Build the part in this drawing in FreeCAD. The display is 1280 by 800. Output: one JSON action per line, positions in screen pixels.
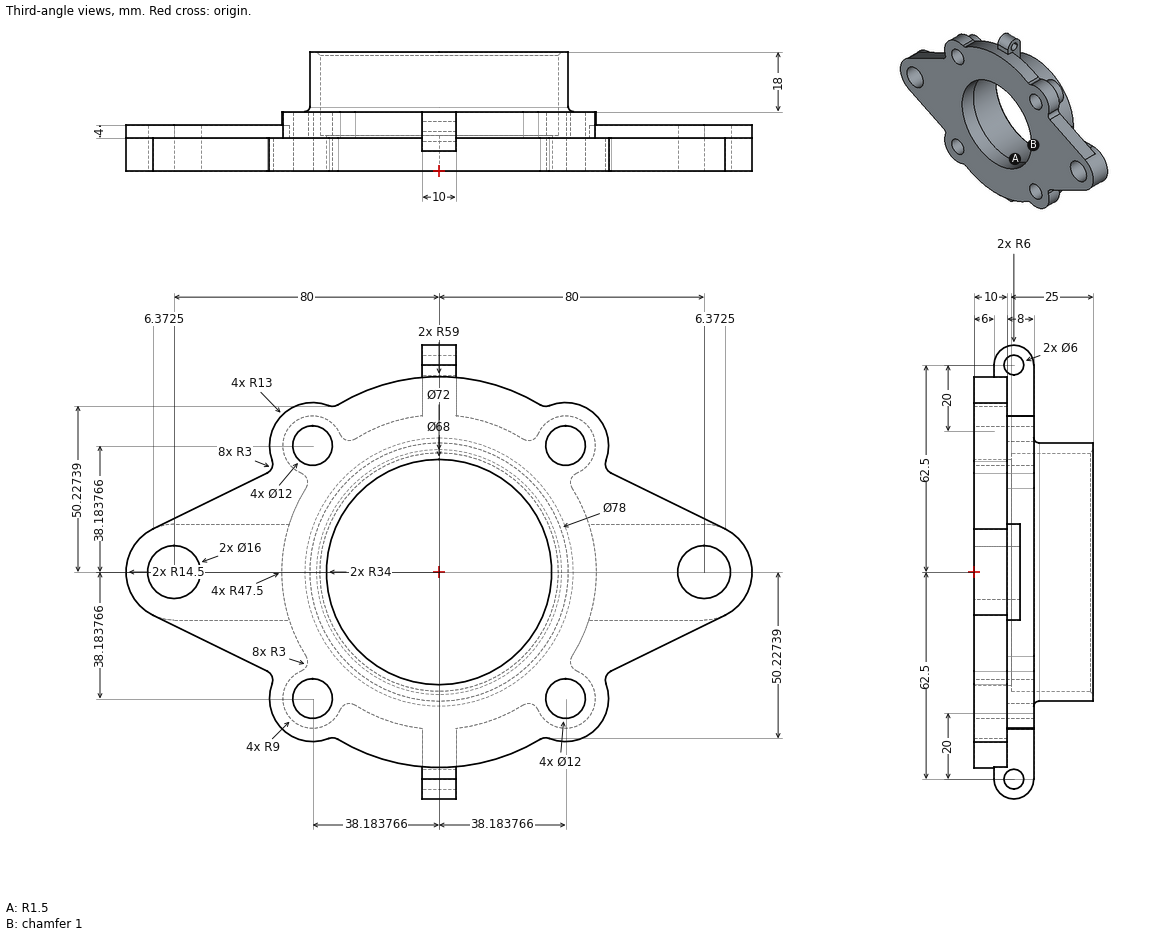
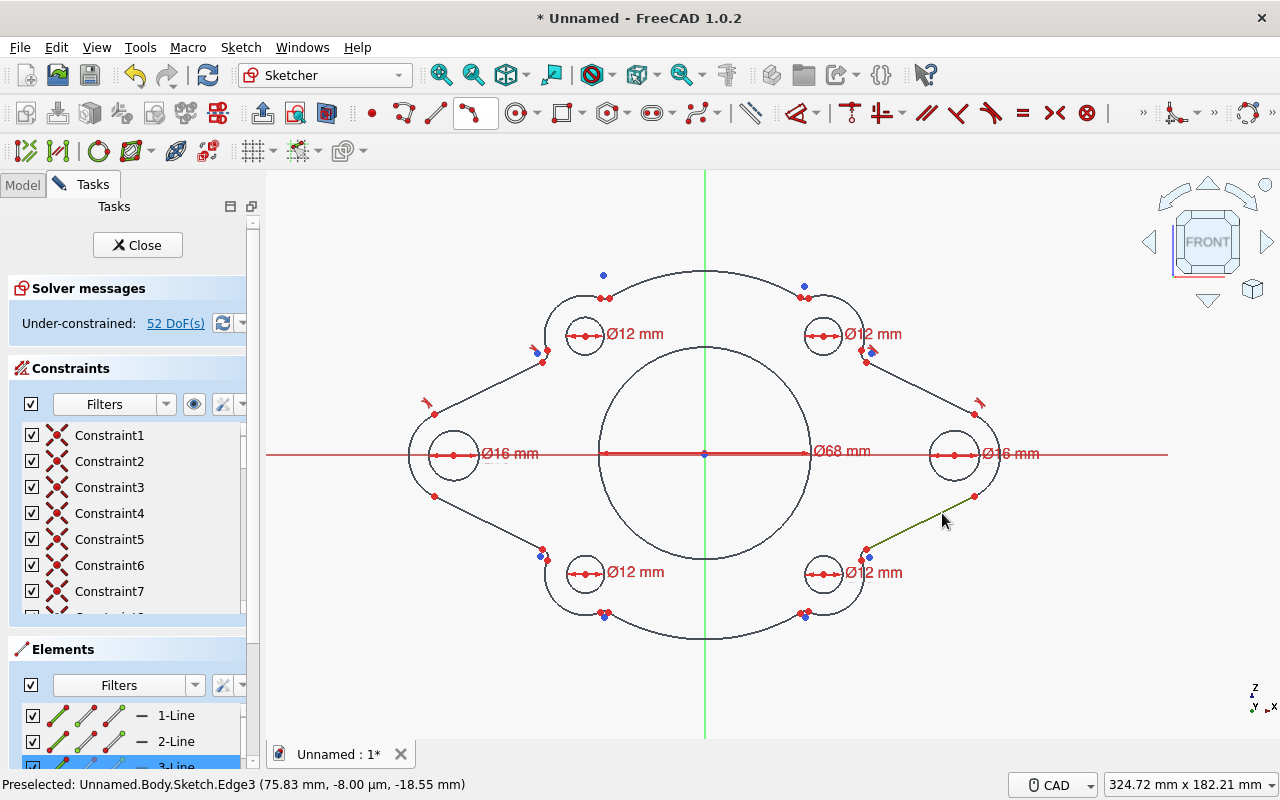
{"action": "left_click", "coordinate": [995, 476]}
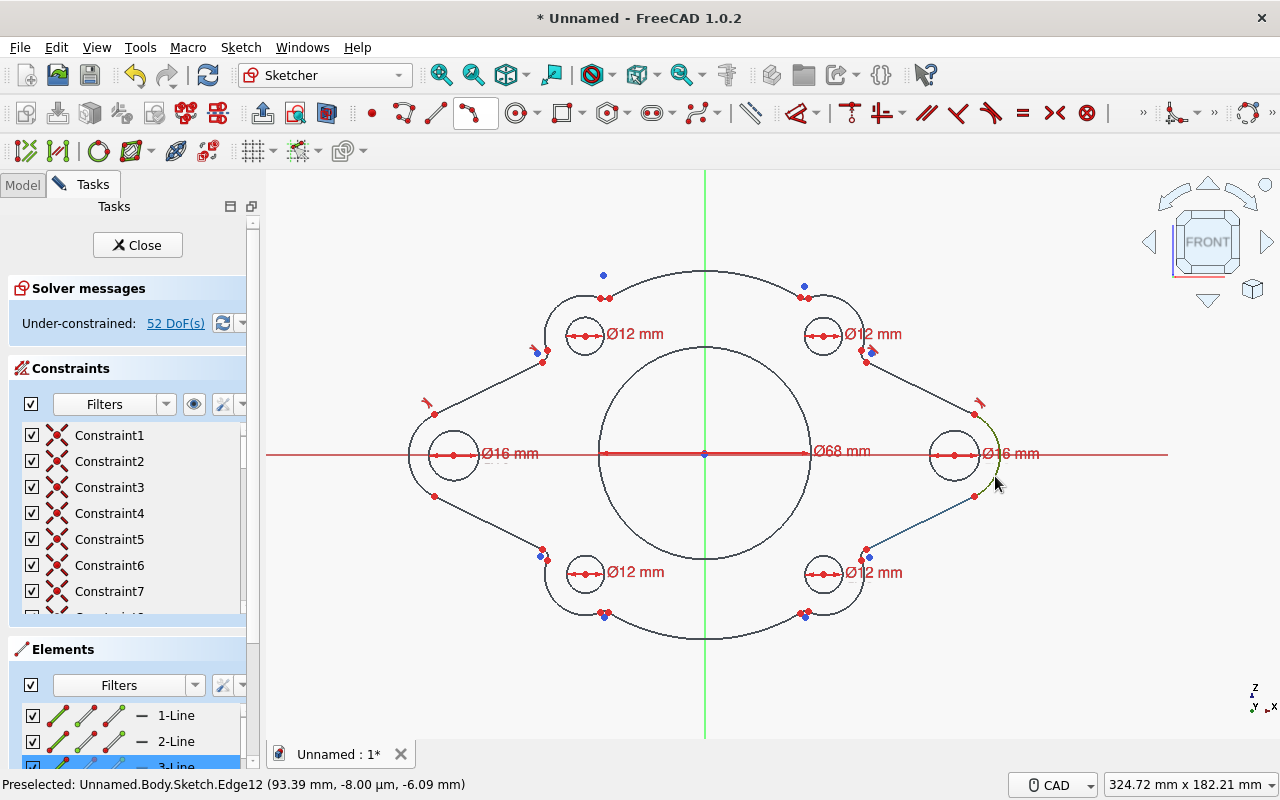
{"action": "left_click", "coordinate": [992, 114]}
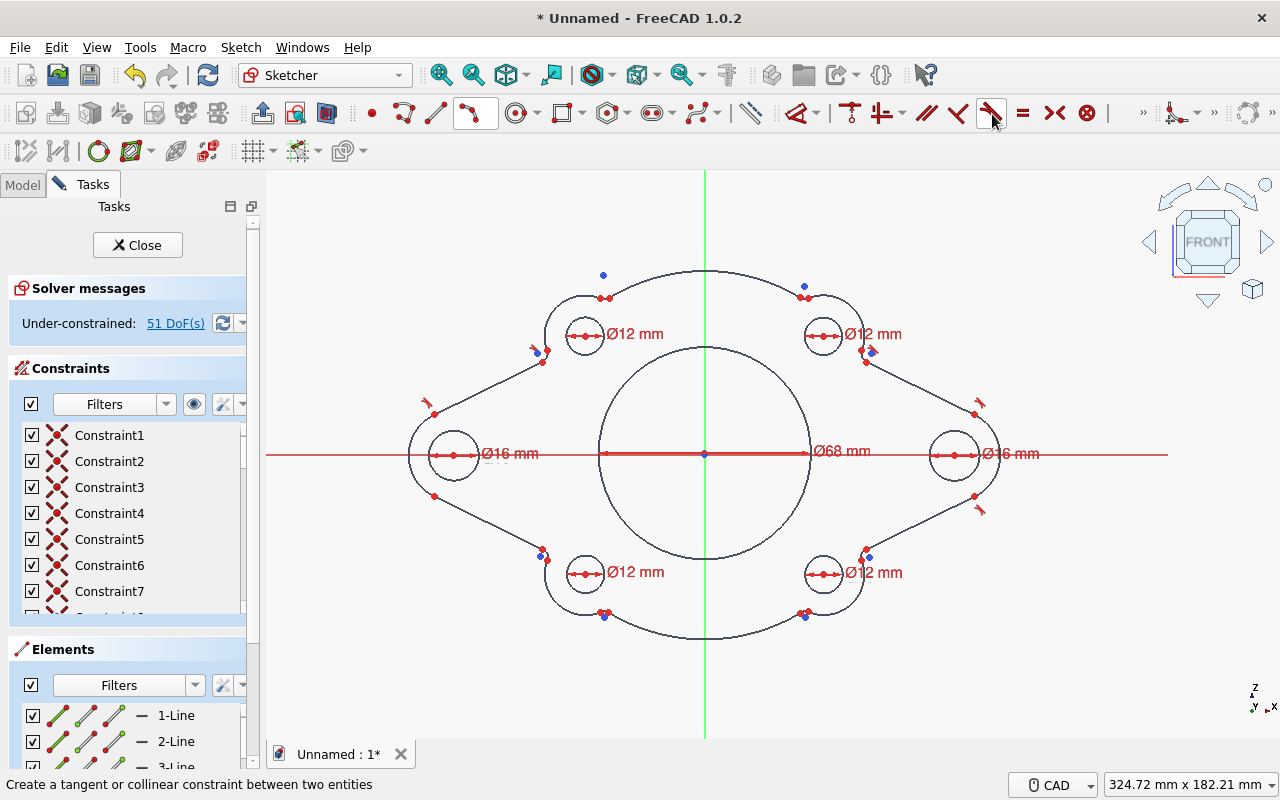
{"action": "left_click", "coordinate": [942, 513]}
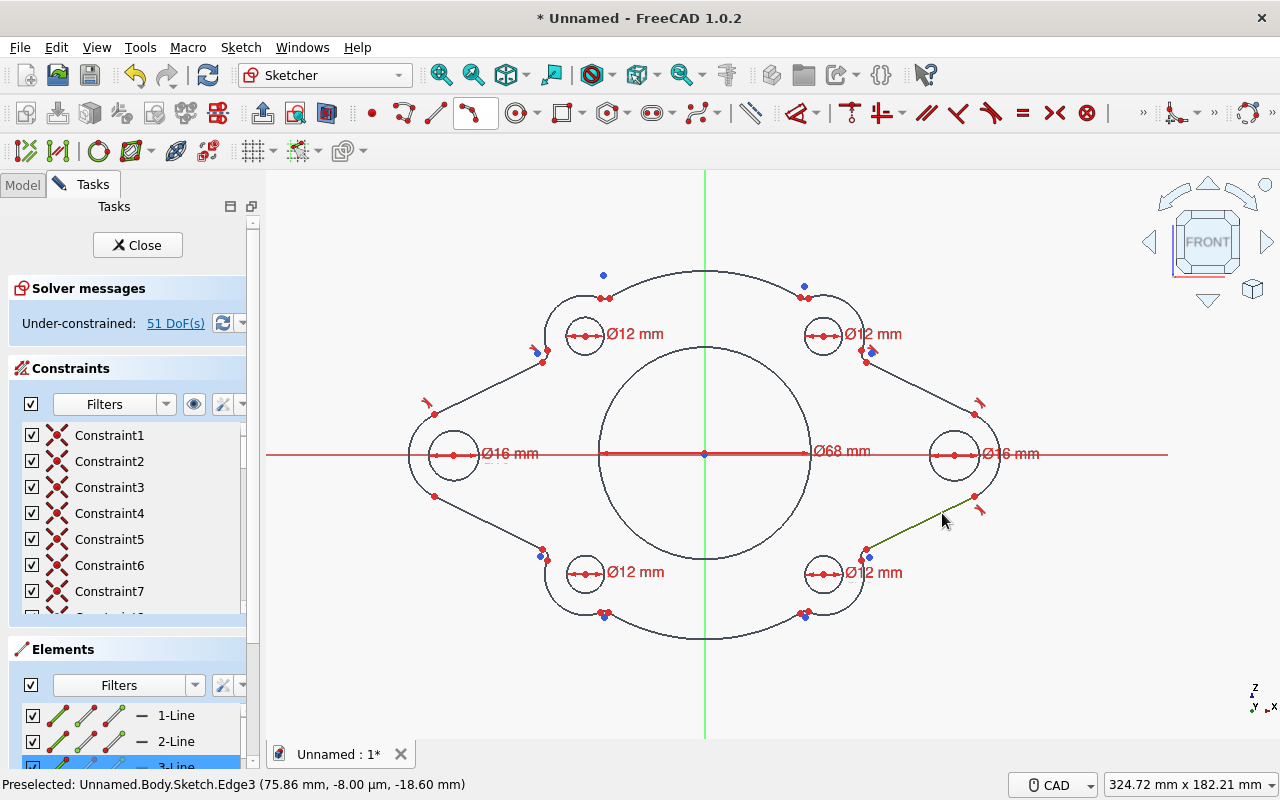
{"action": "scroll", "coordinate": [862, 554], "scroll_direction": "up", "scroll_amount": 4}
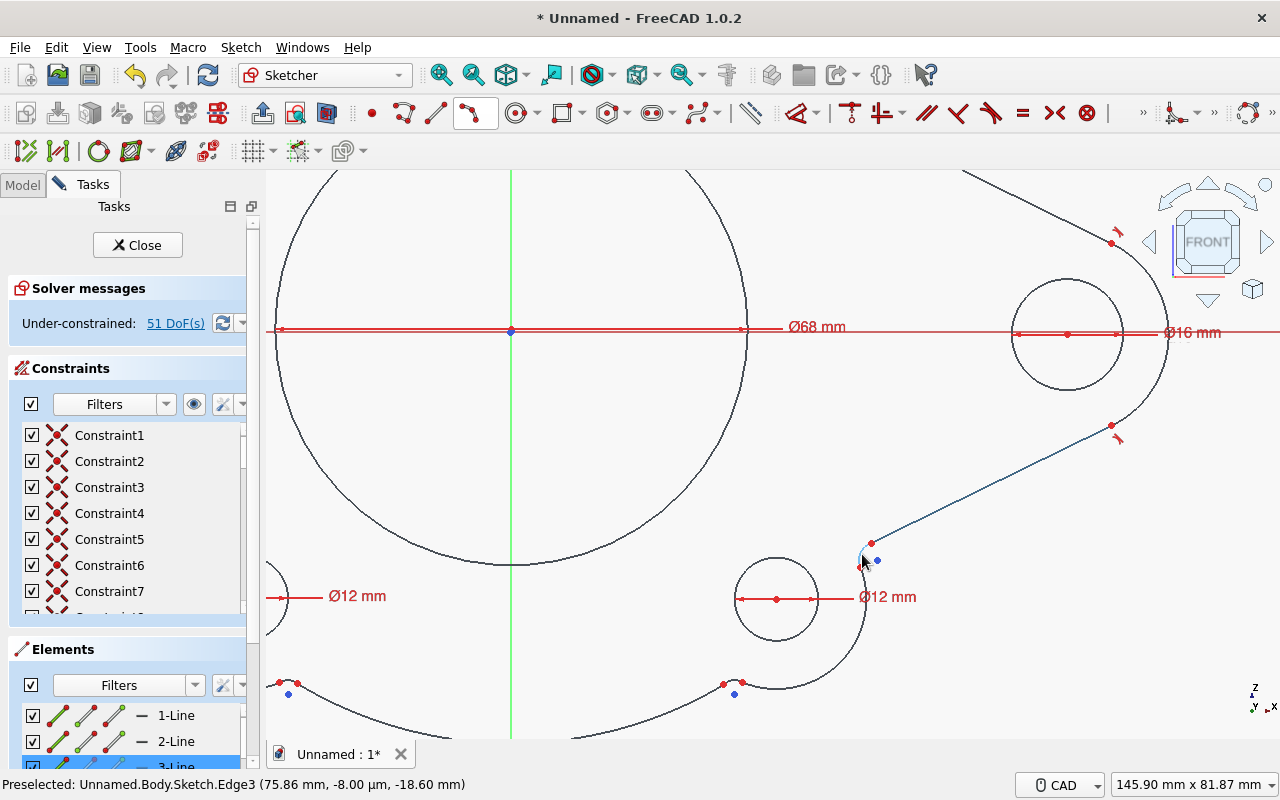
{"action": "left_click", "coordinate": [861, 553]}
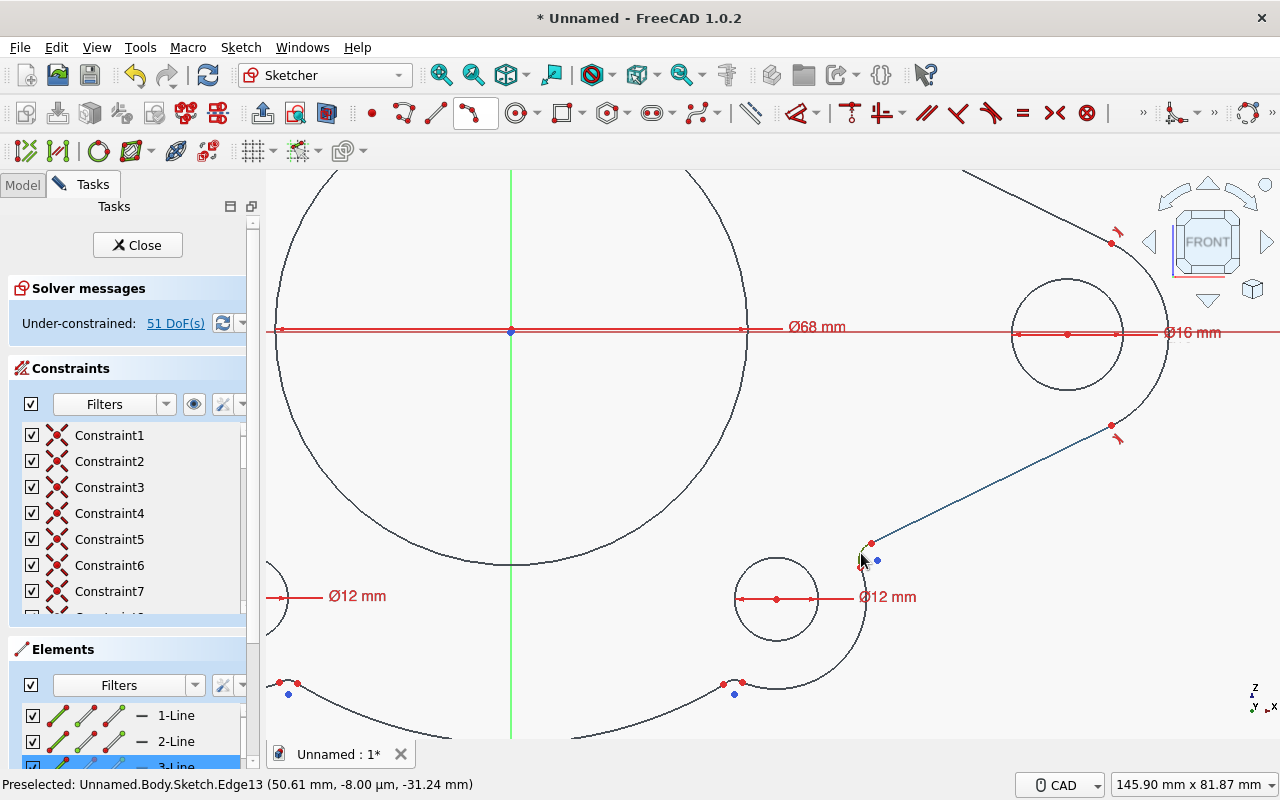
{"action": "left_click", "coordinate": [992, 114]}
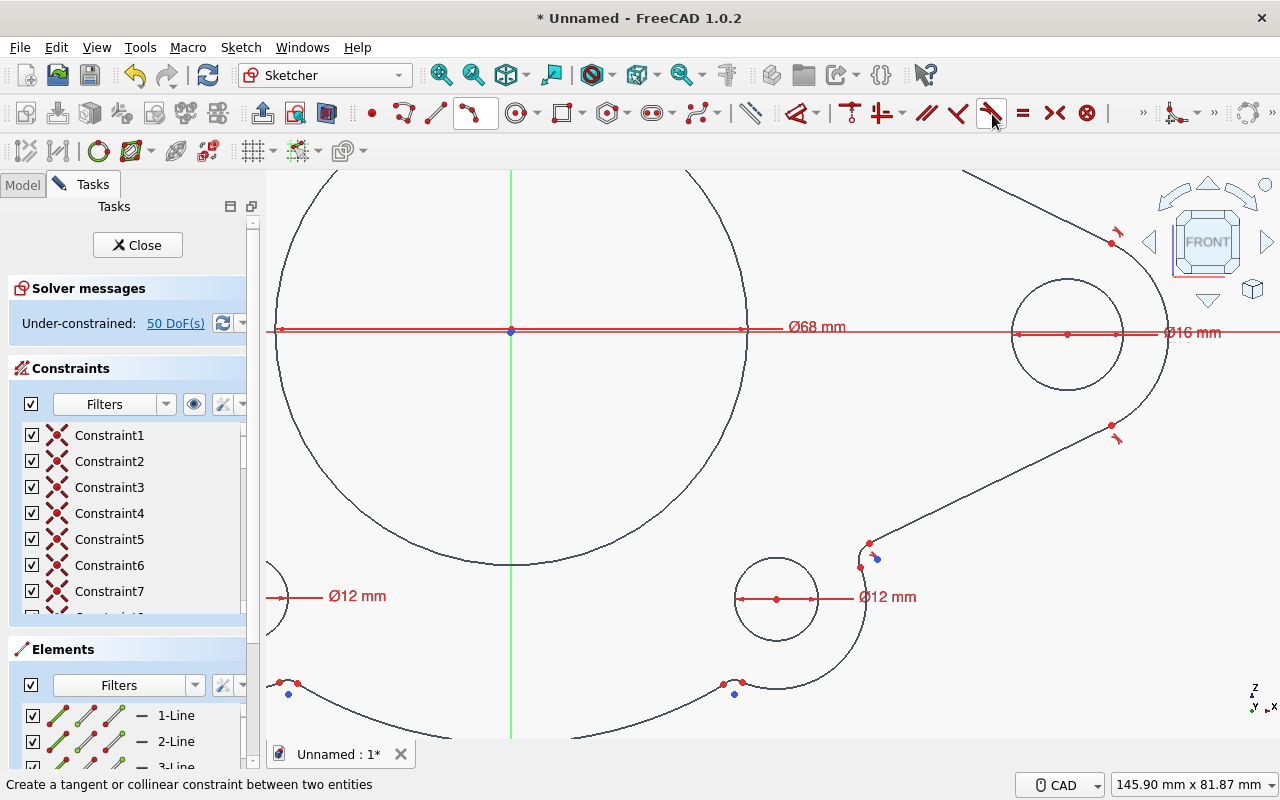
{"action": "scroll", "coordinate": [862, 554], "scroll_direction": "down", "scroll_amount": 4}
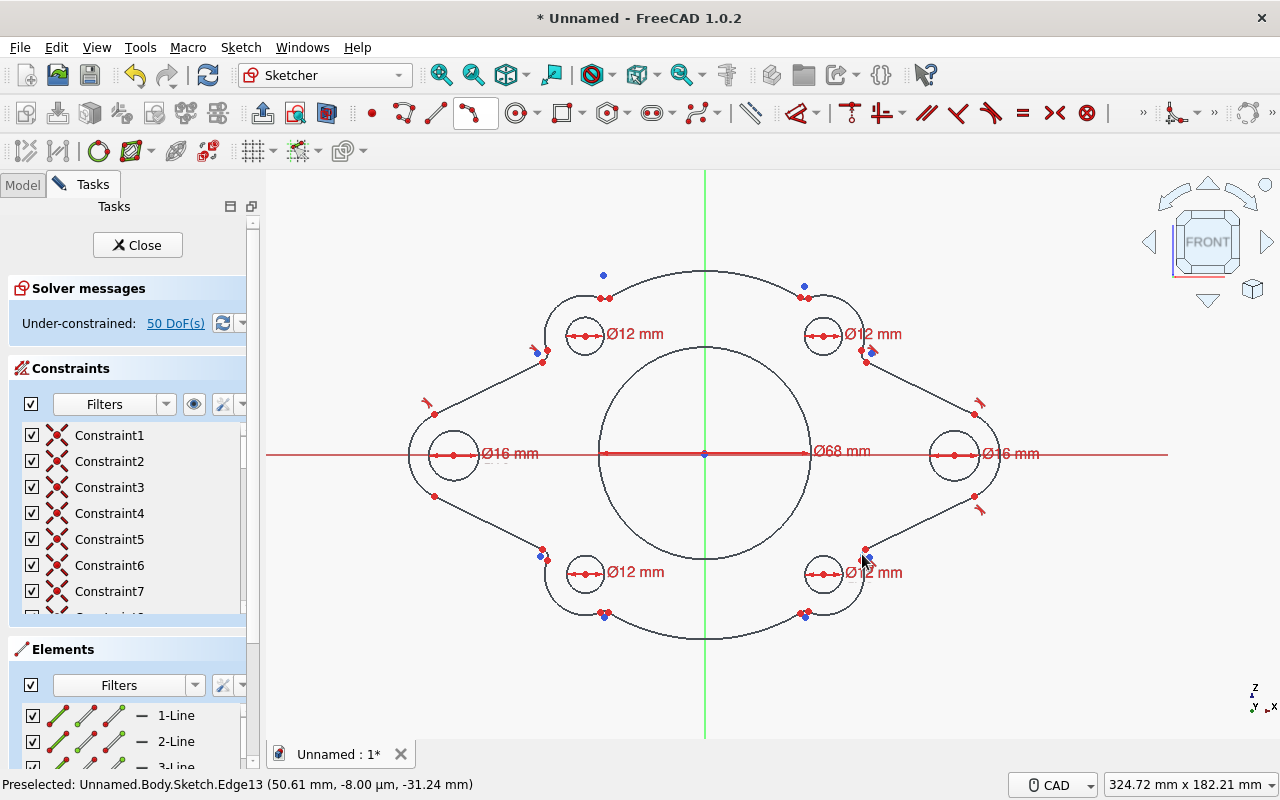
{"action": "left_click", "coordinate": [510, 534]}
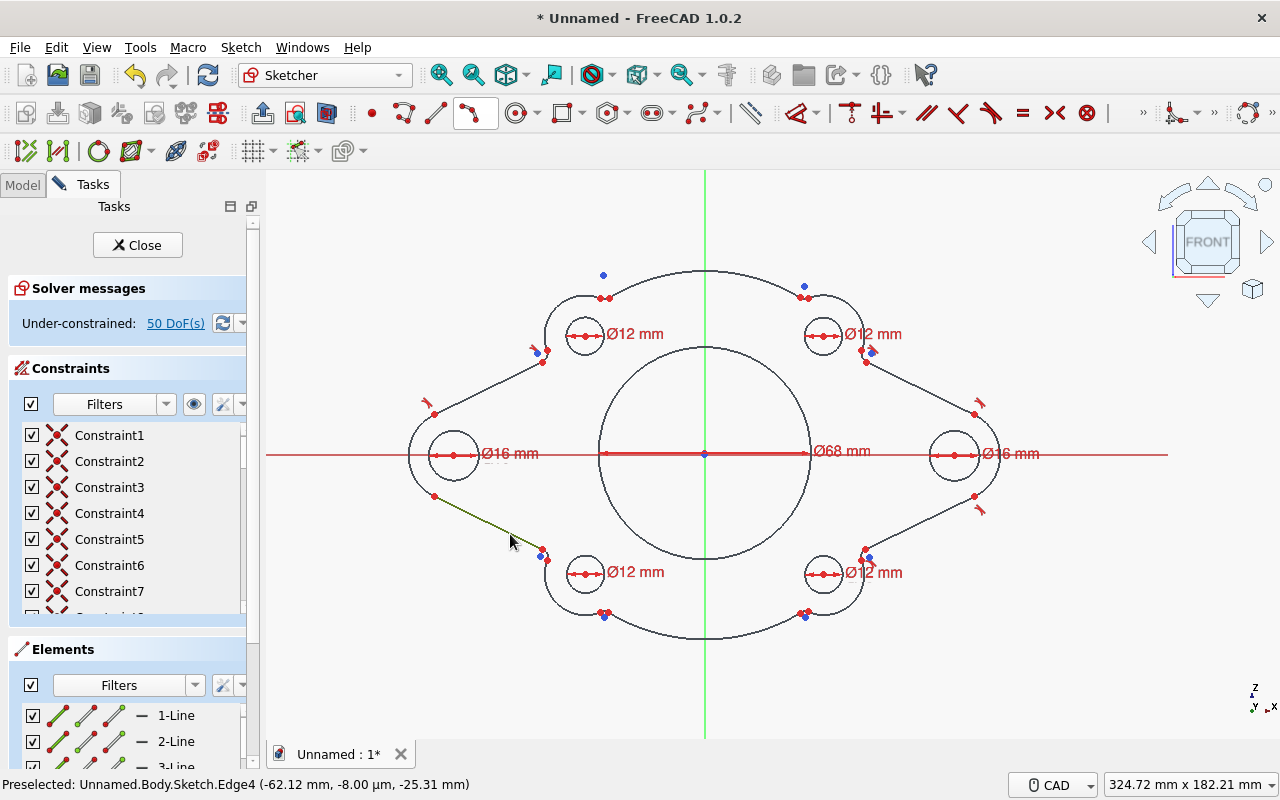
{"action": "scroll", "coordinate": [547, 554], "scroll_direction": "up", "scroll_amount": 4}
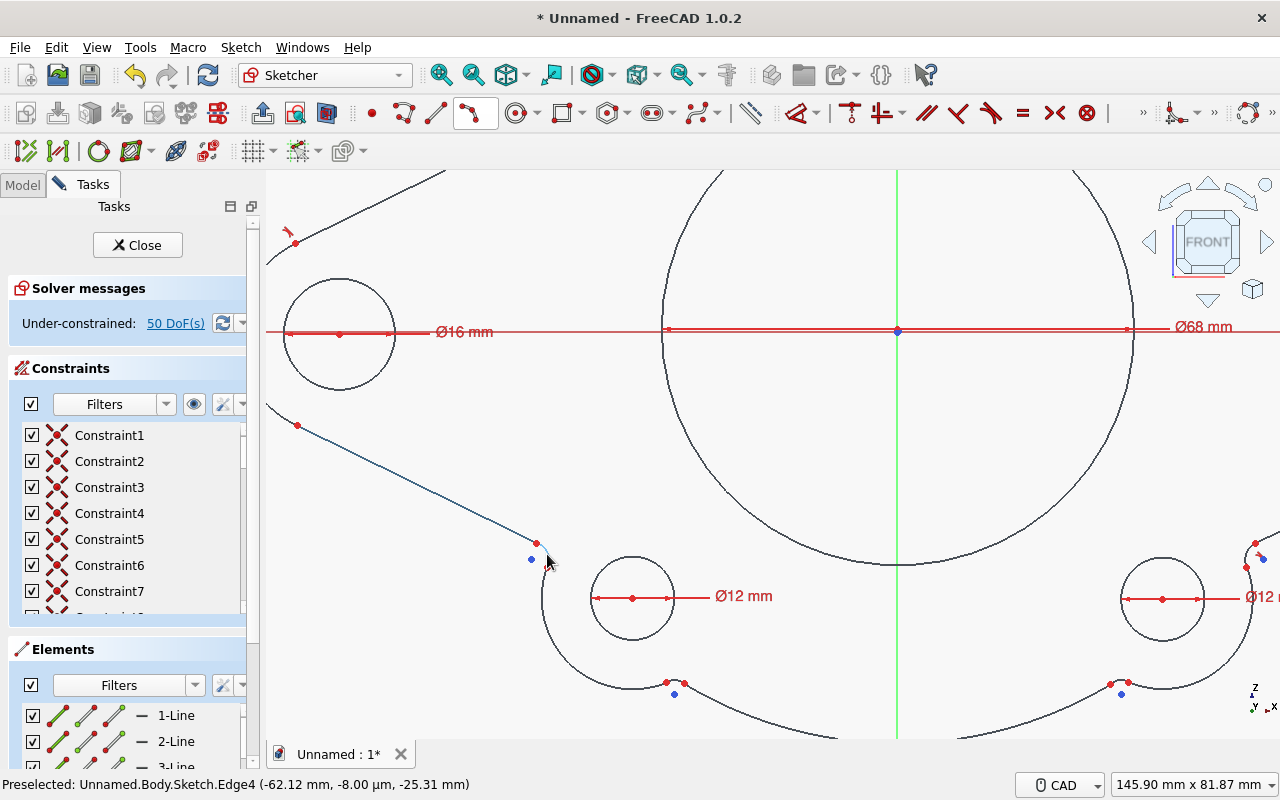
{"action": "left_click", "coordinate": [548, 553]}